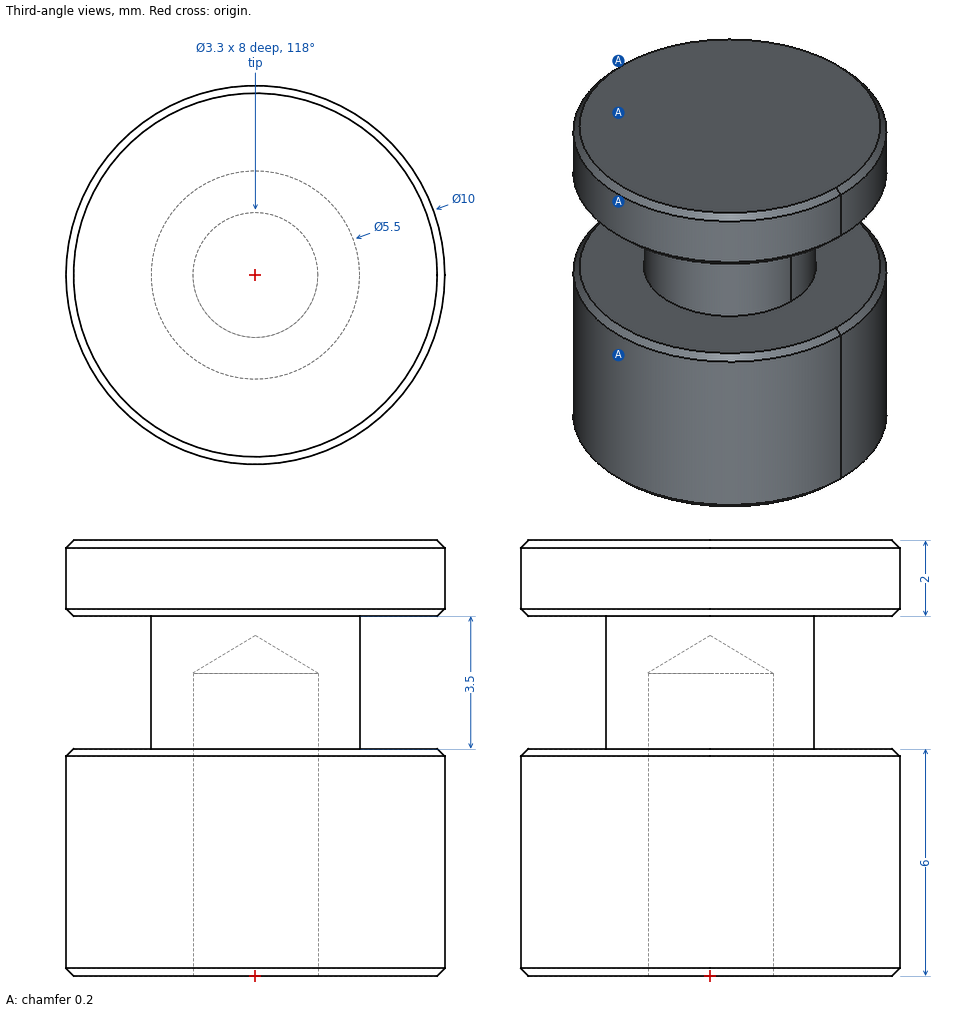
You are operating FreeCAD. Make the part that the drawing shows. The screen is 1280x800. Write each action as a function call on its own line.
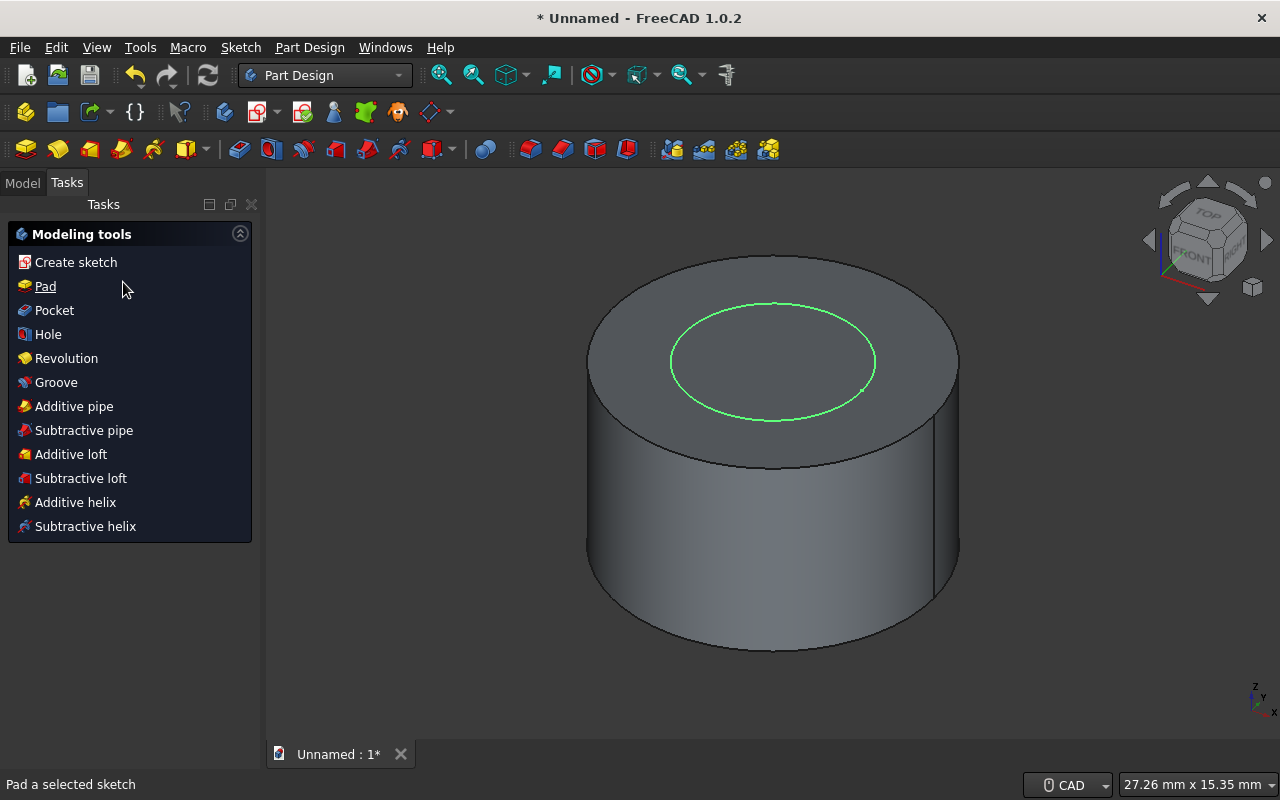
click(26, 150)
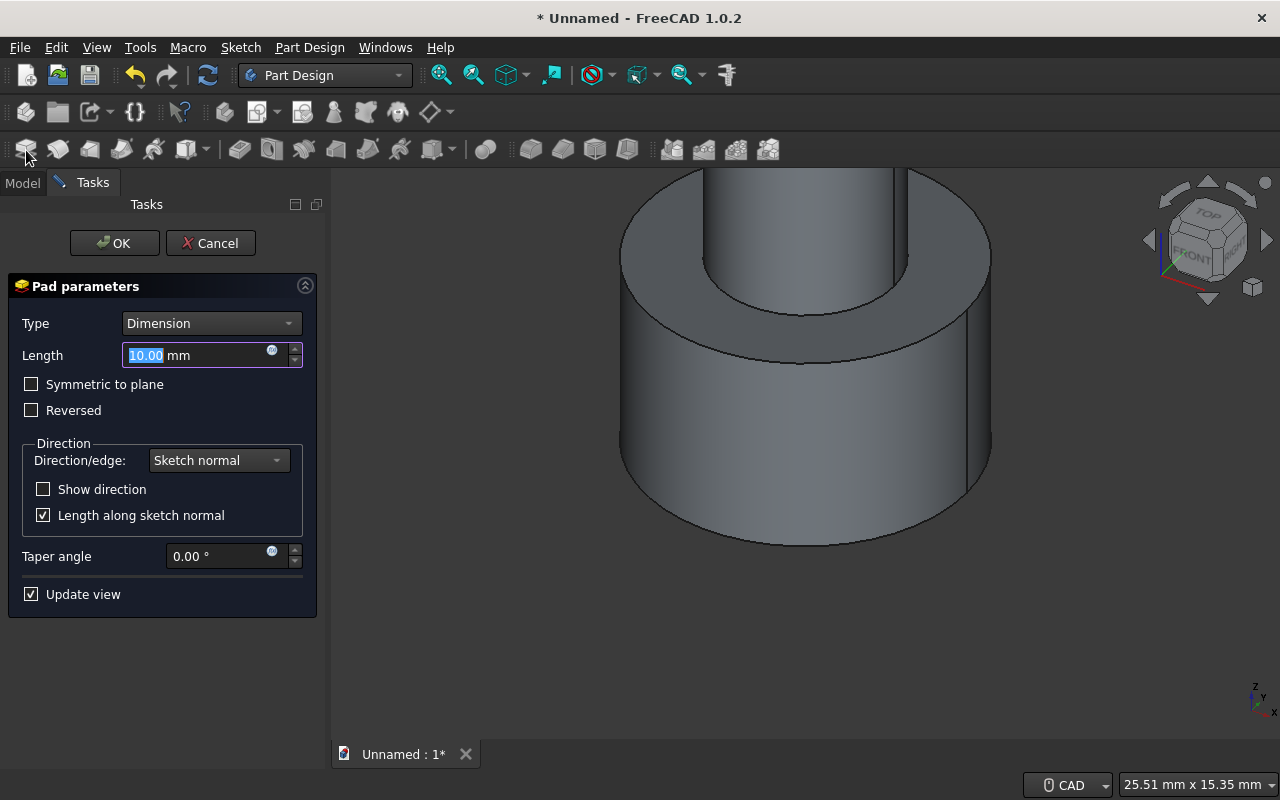
text(3.5)
key(Tab)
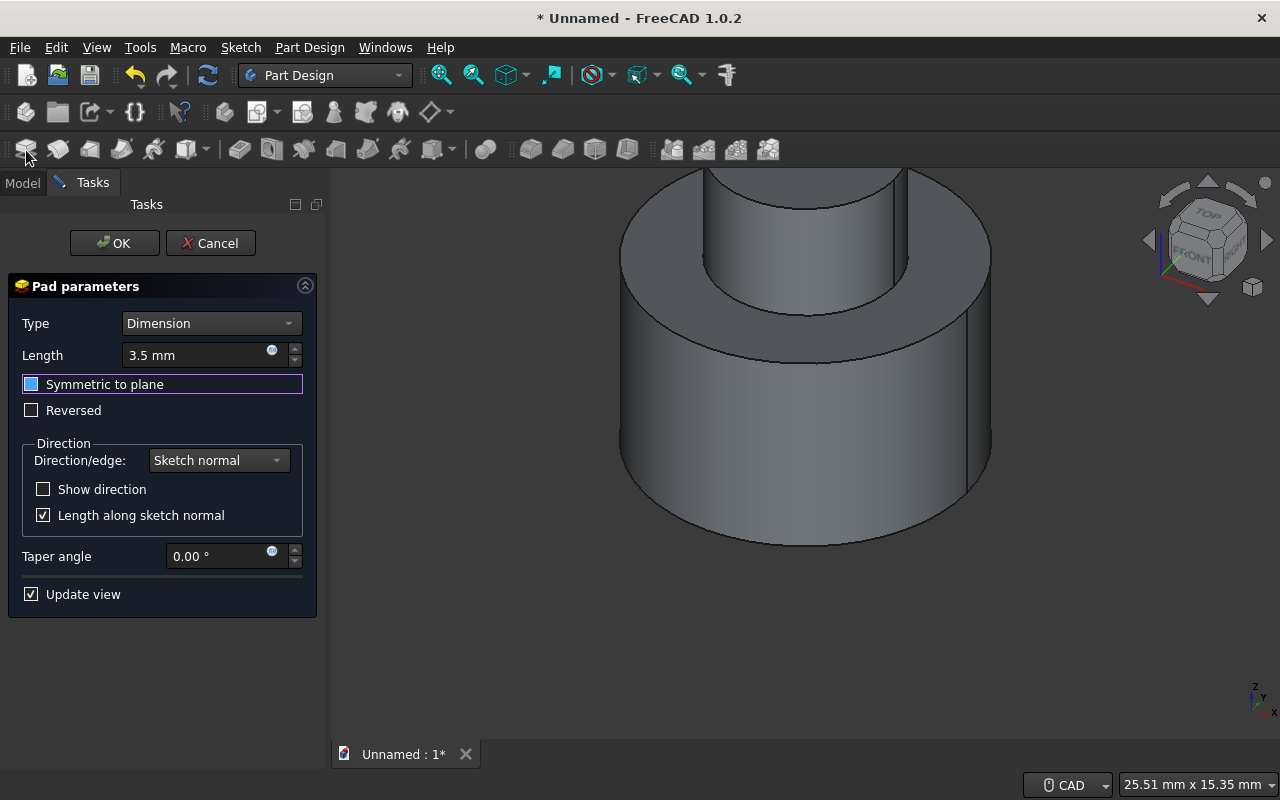
click(115, 243)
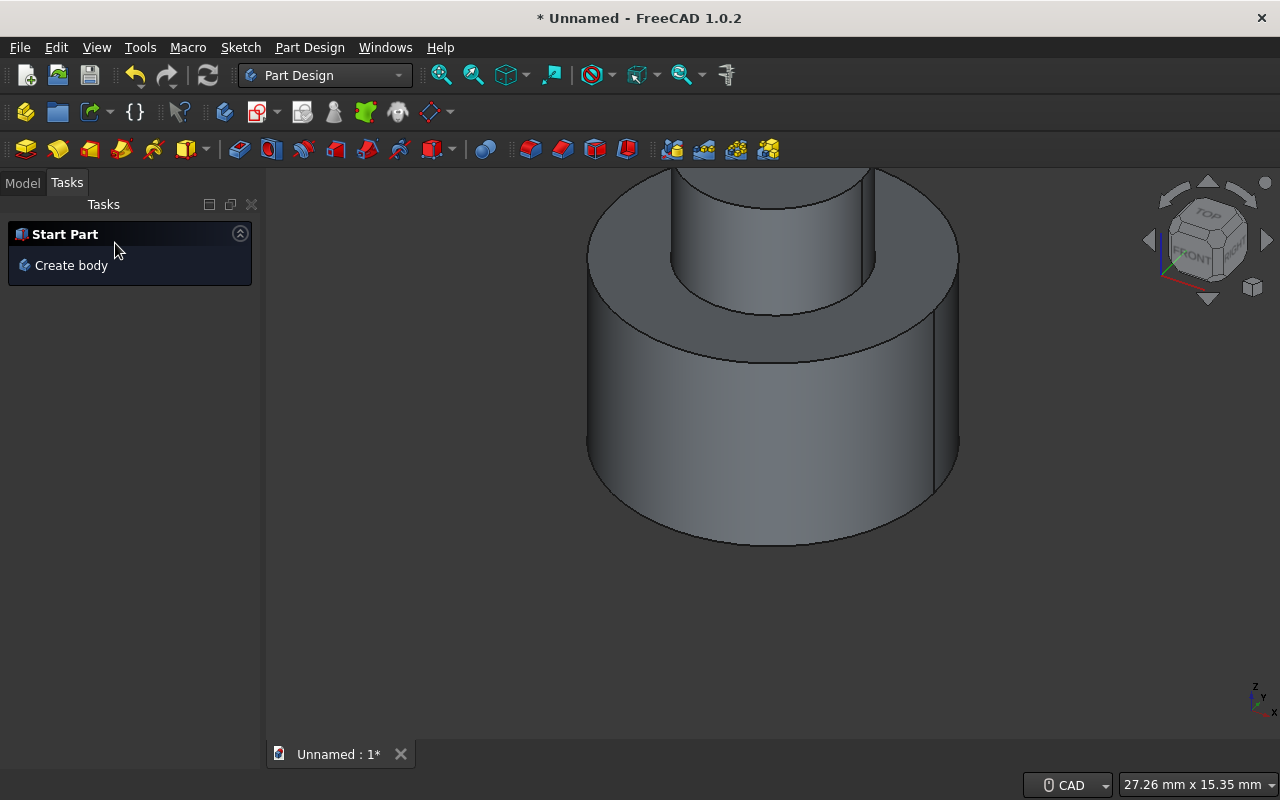
click(442, 76)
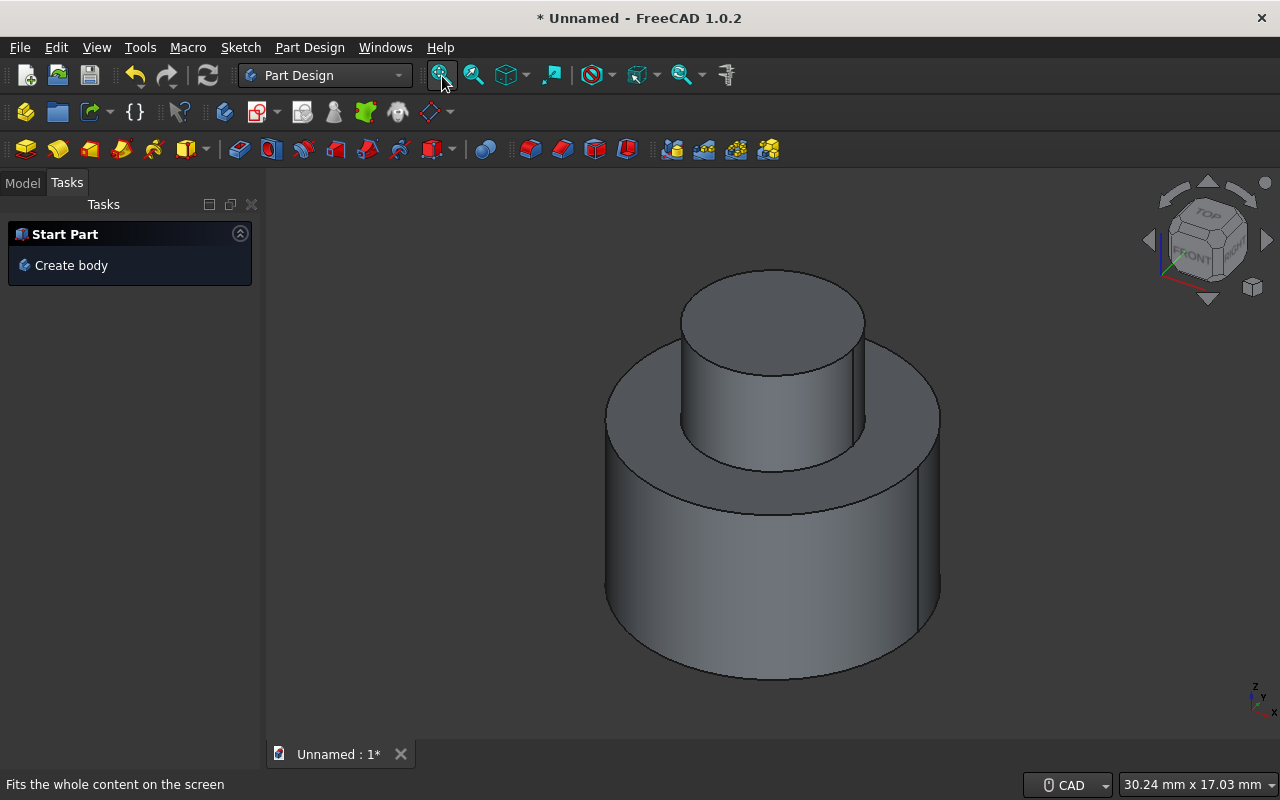
click(773, 322)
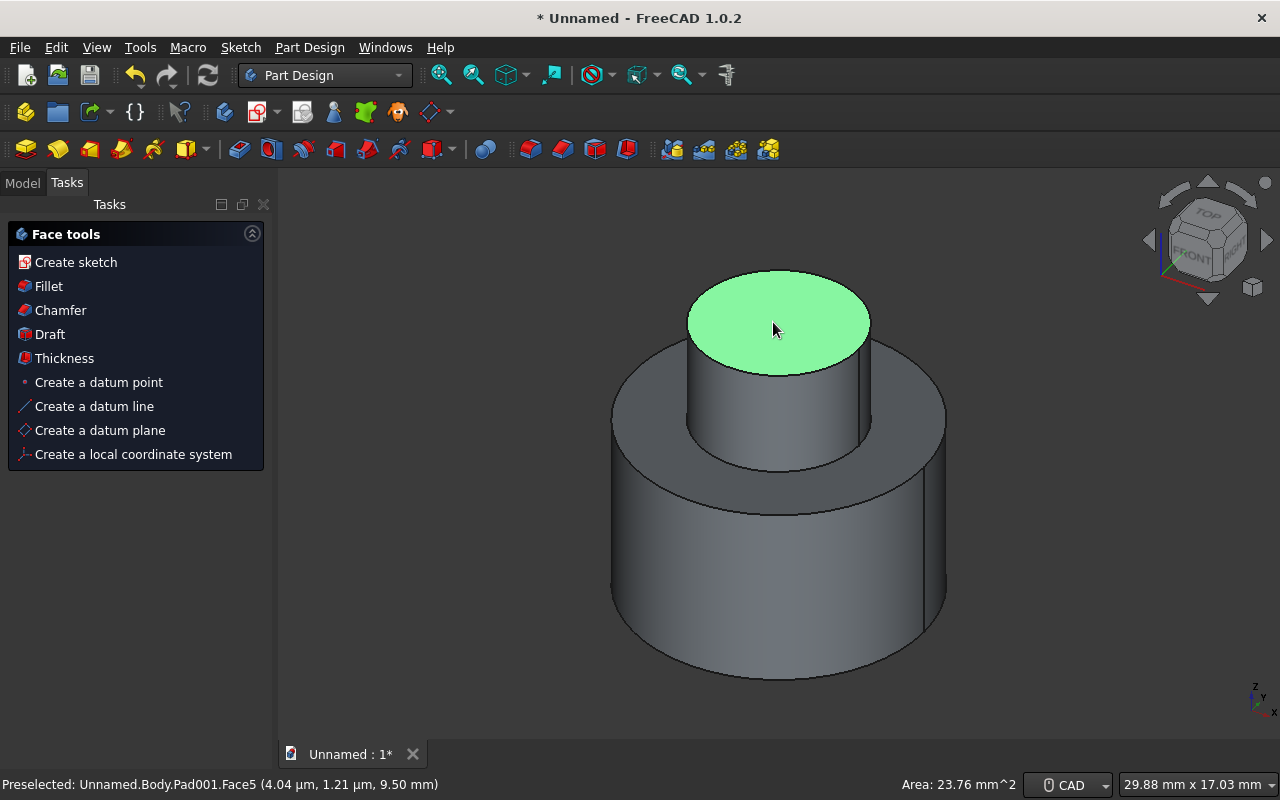
click(258, 112)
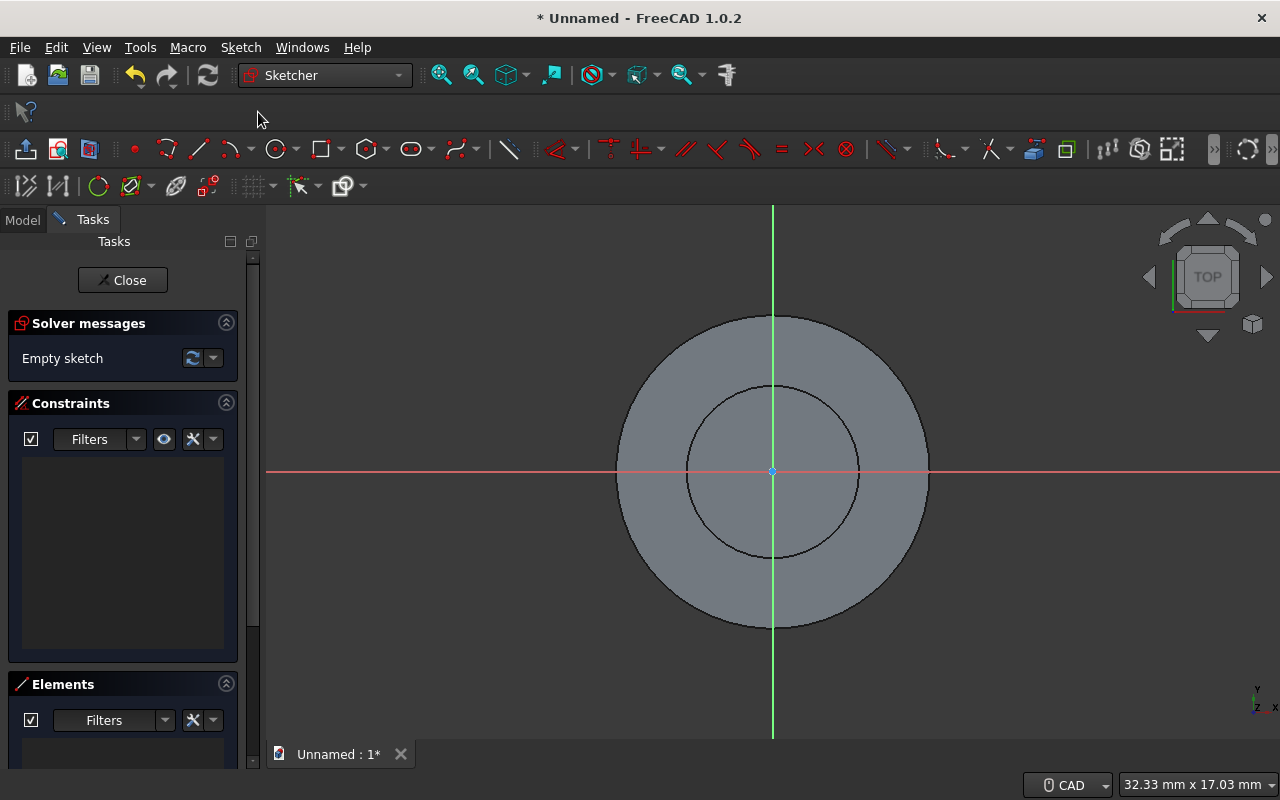
click(276, 150)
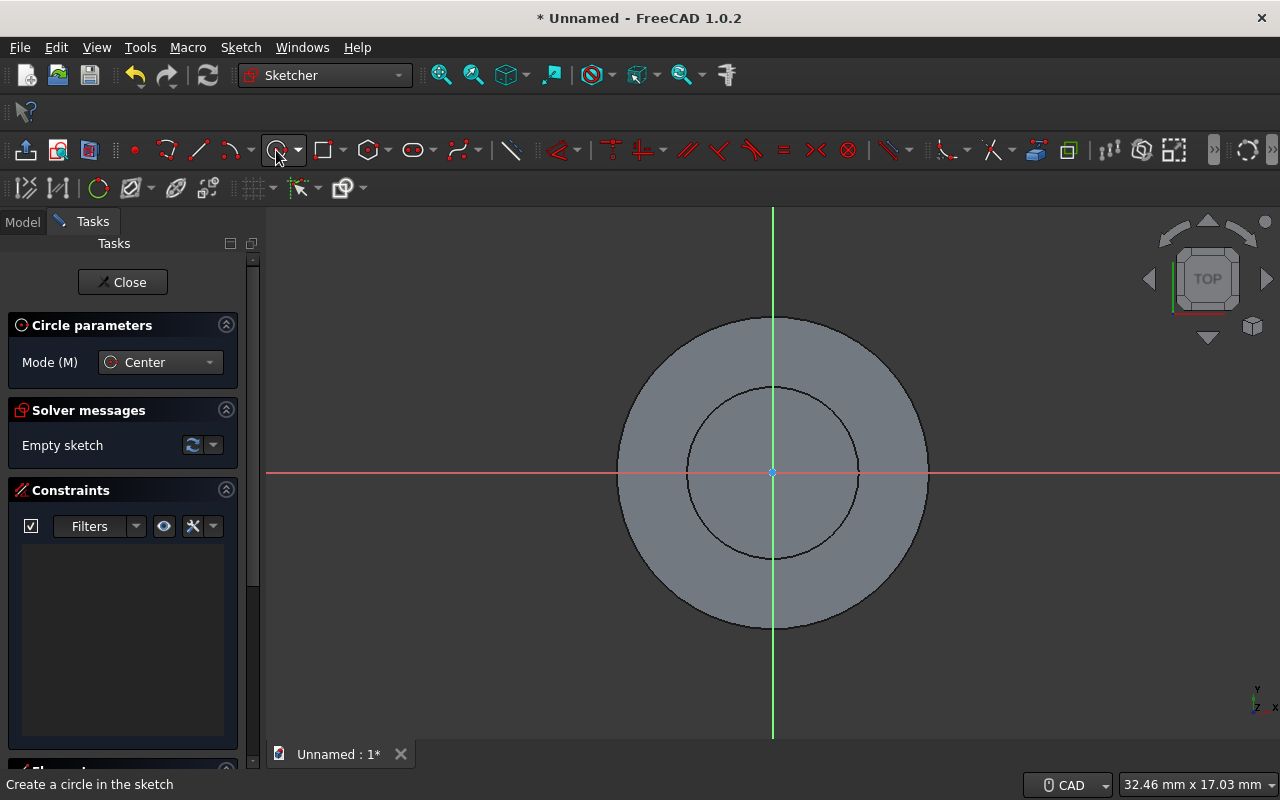
click(773, 473)
move(883, 363)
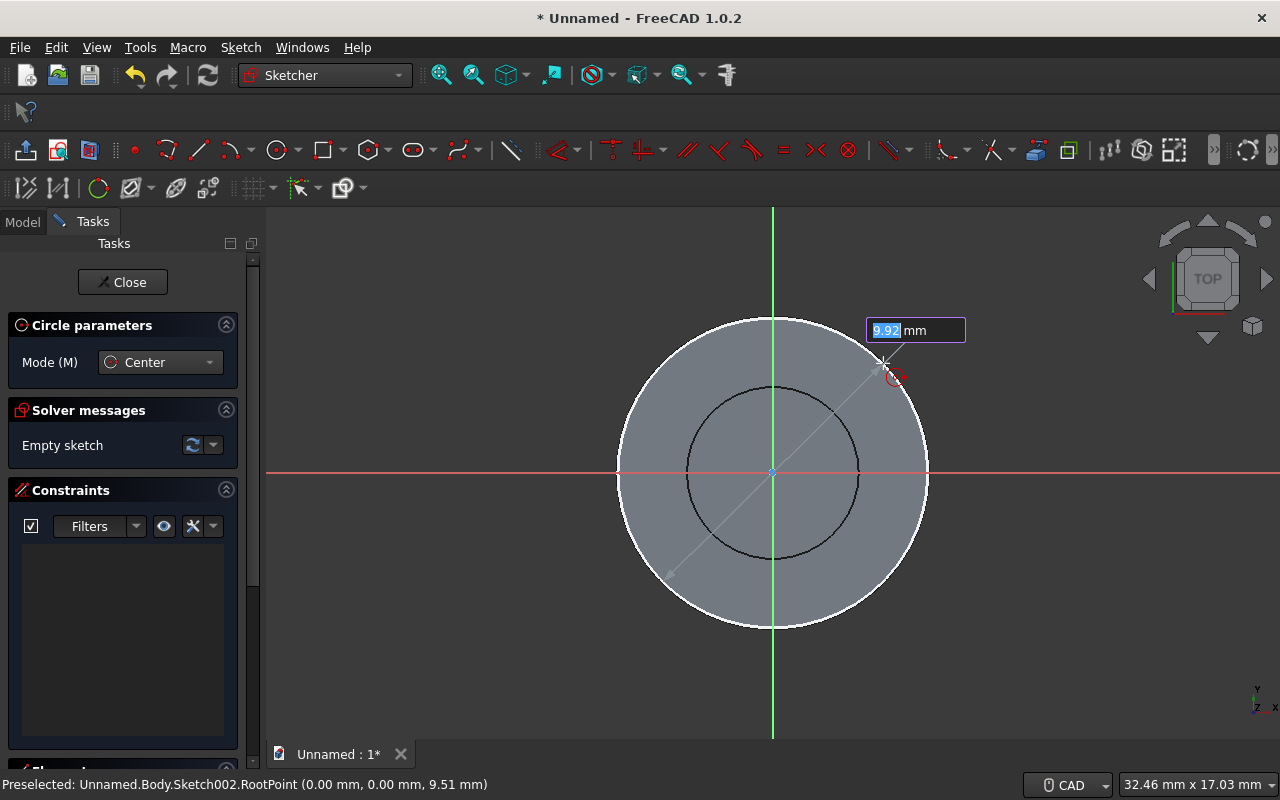
text(10)
key(Return)
key(Escape)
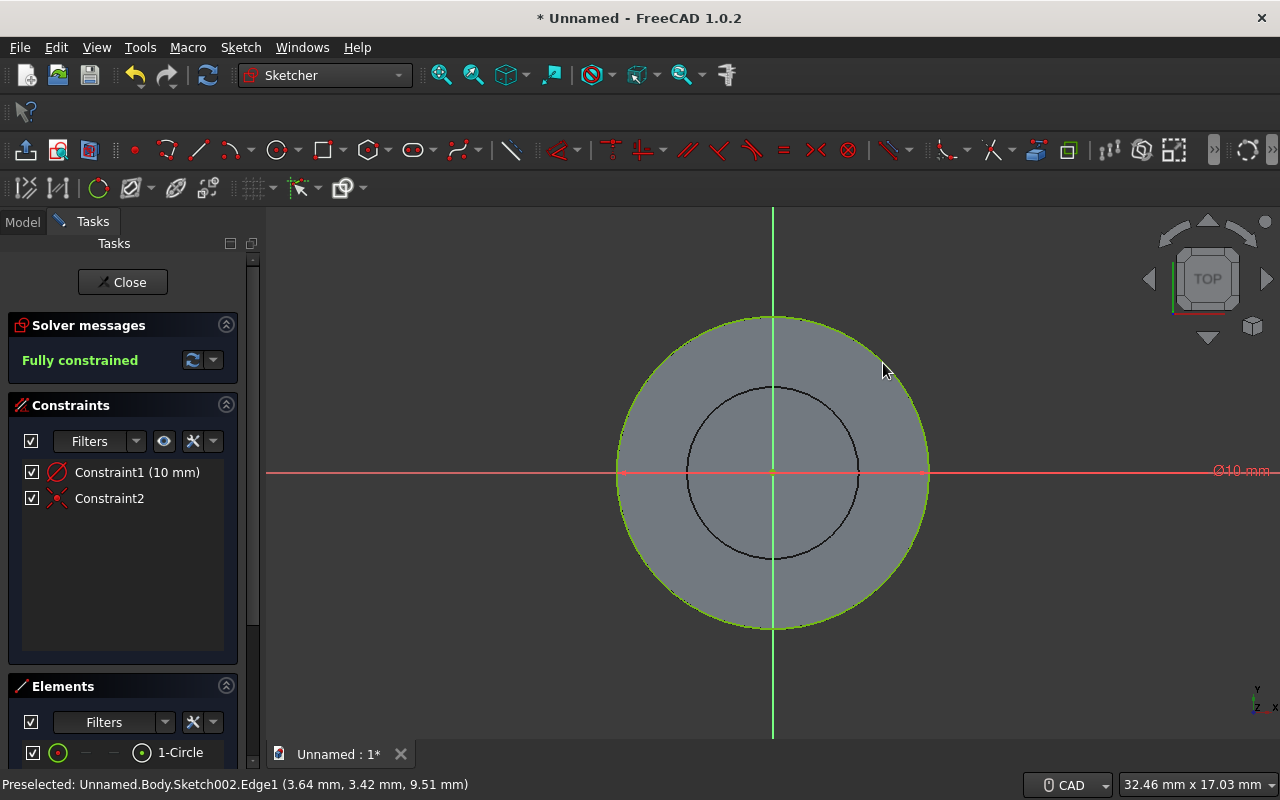
click(123, 282)